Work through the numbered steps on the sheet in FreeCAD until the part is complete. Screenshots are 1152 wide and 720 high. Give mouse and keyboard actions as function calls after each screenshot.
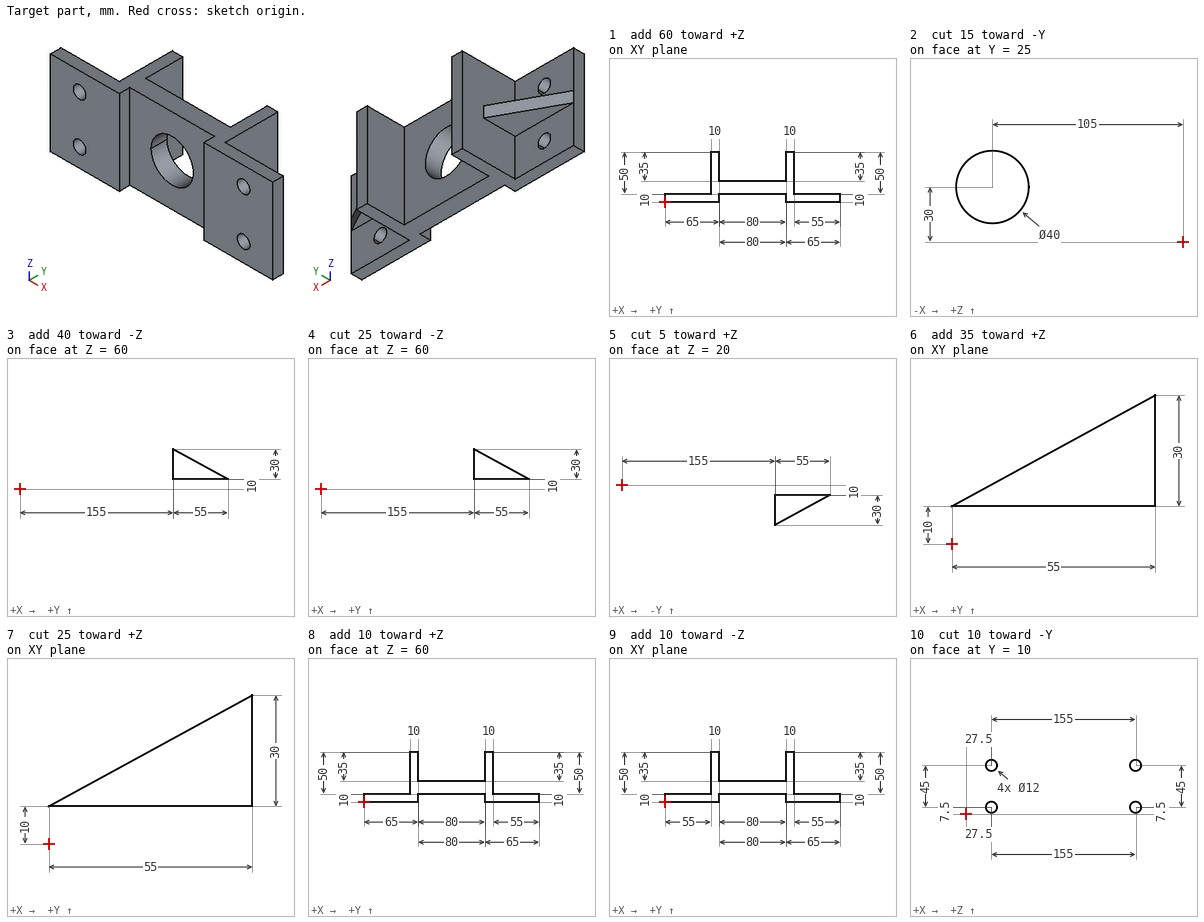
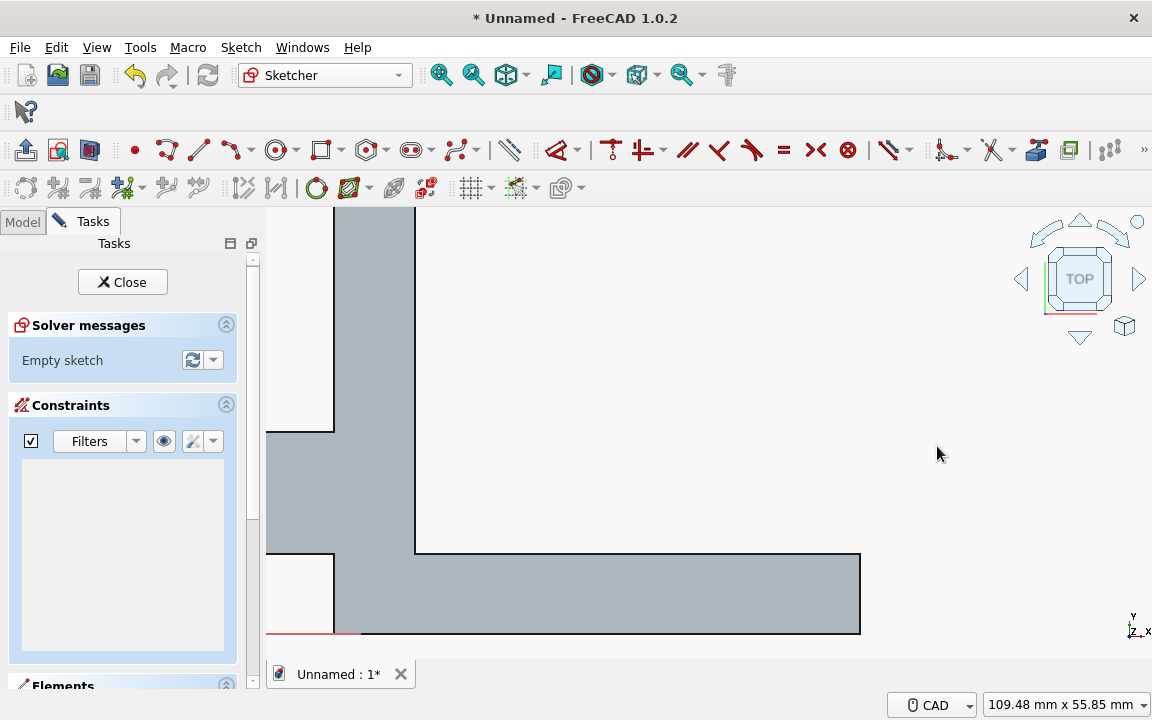
key(g)
key(m)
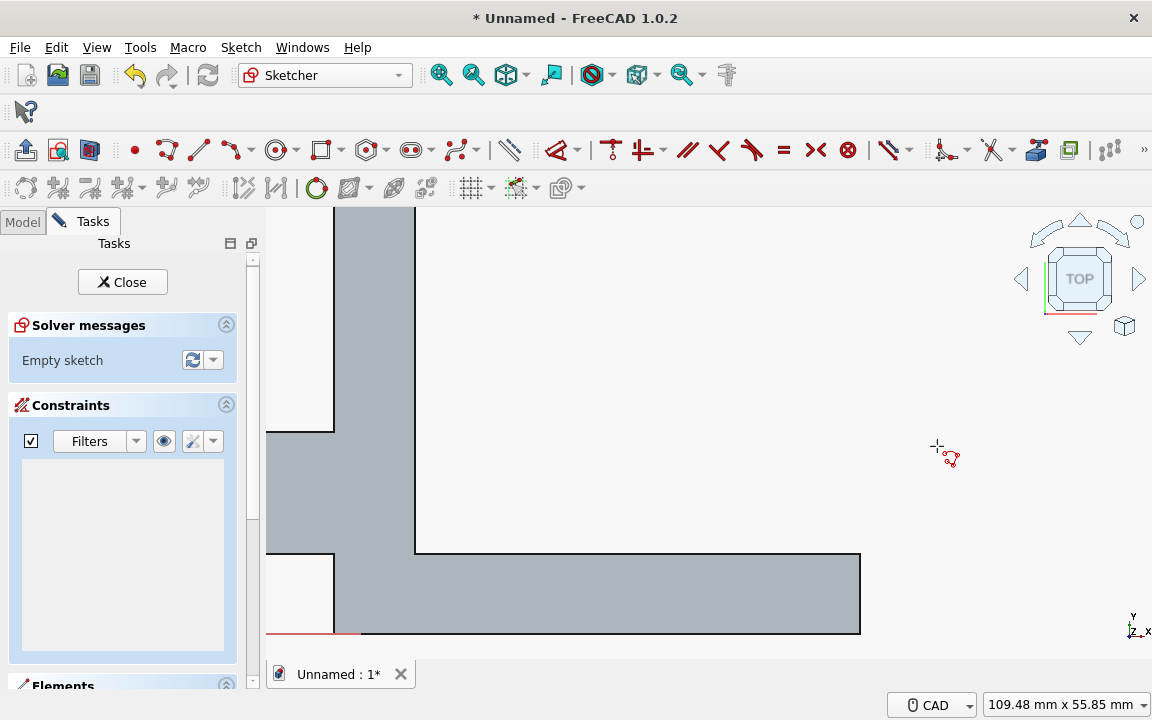
click(415, 554)
click(860, 554)
click(415, 311)
click(415, 555)
key(Escape)
key(Escape)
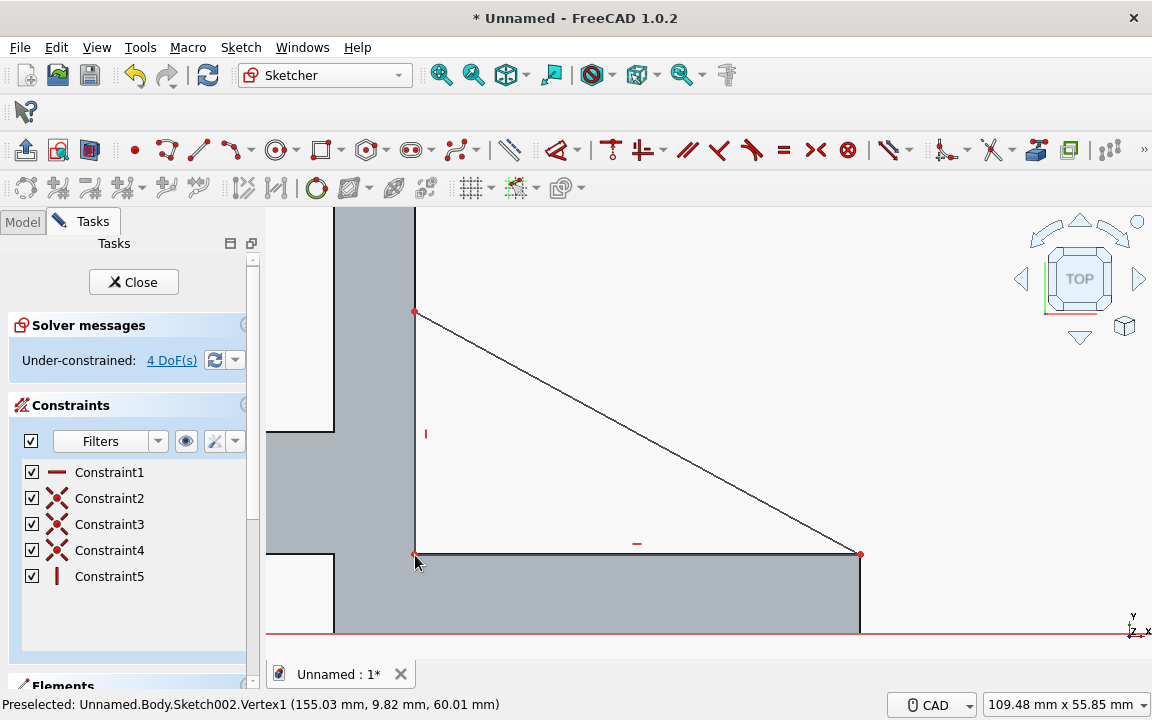
key(d)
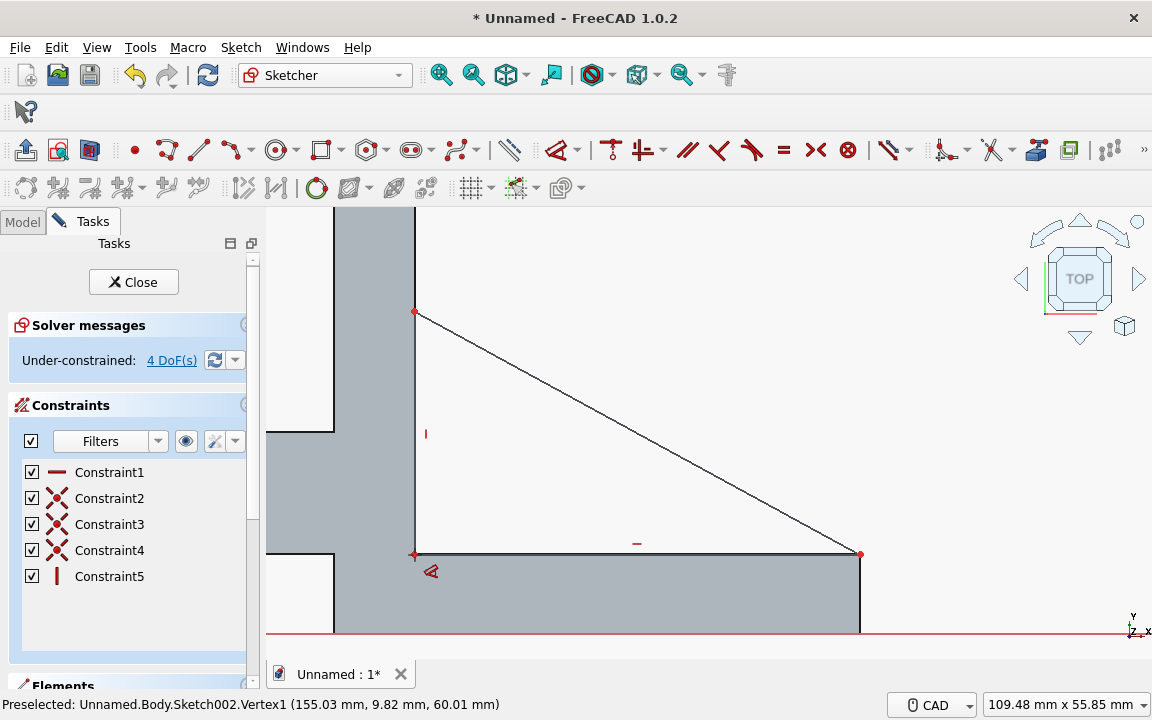
click(548, 555)
click(637, 589)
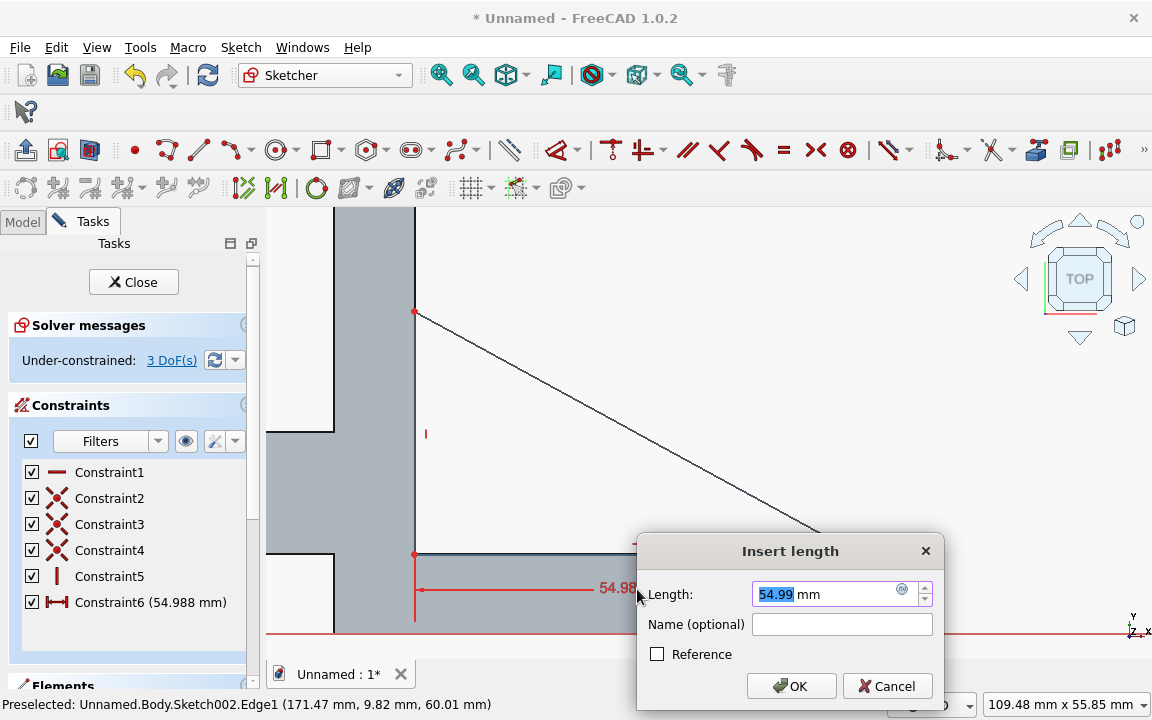
text(55)
key(Return)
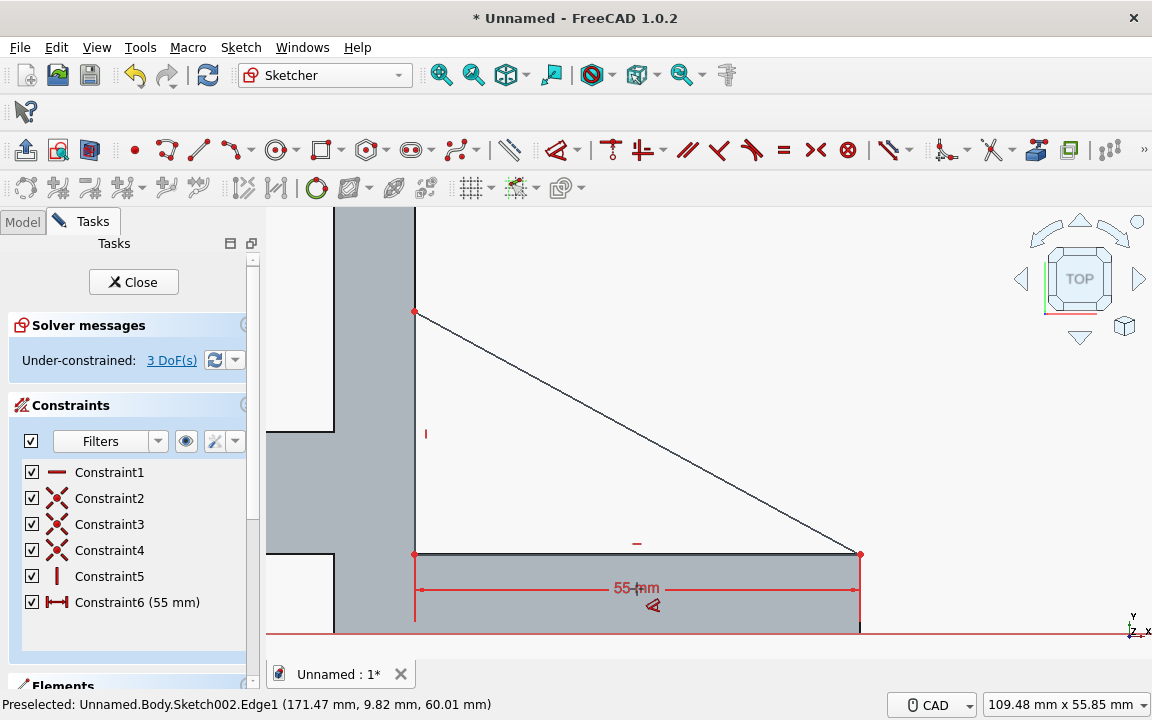
click(415, 385)
click(381, 433)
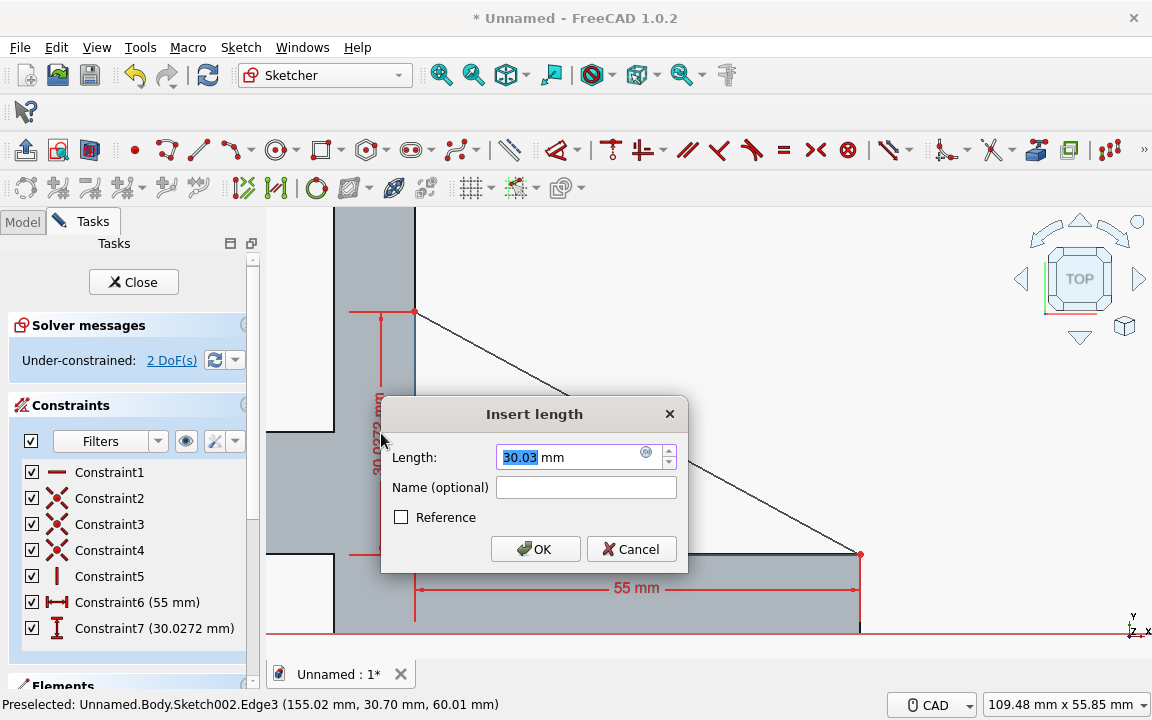
text(30)
key(Return)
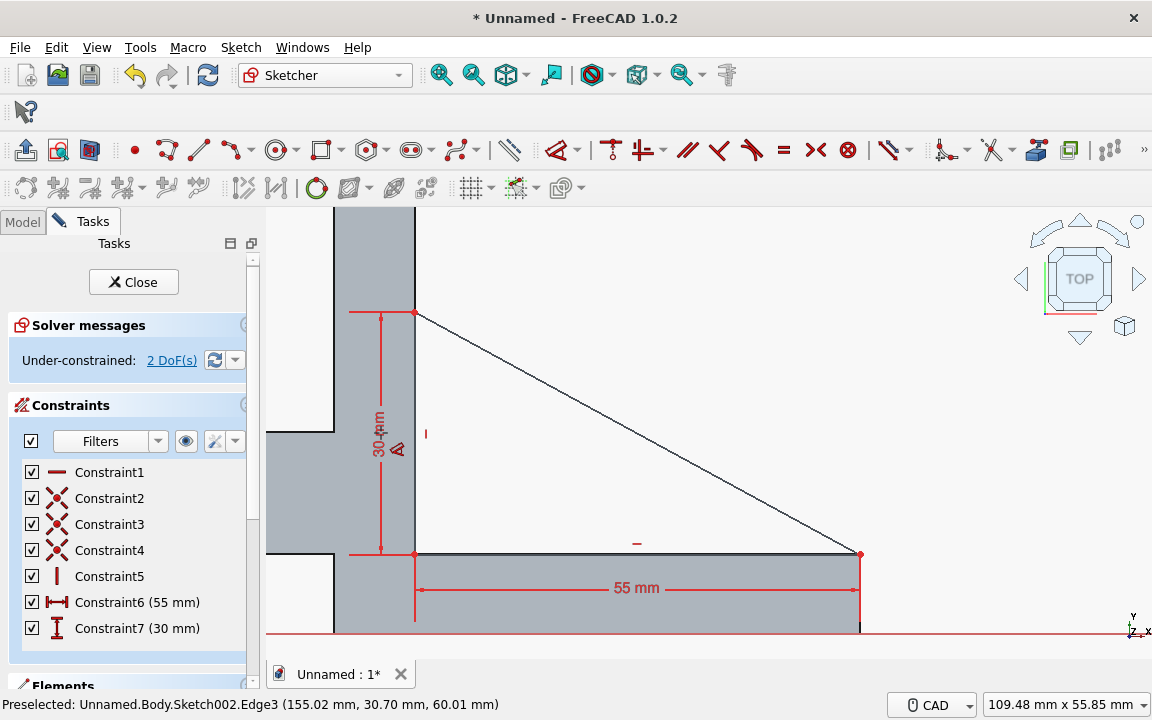
click(415, 555)
click(449, 593)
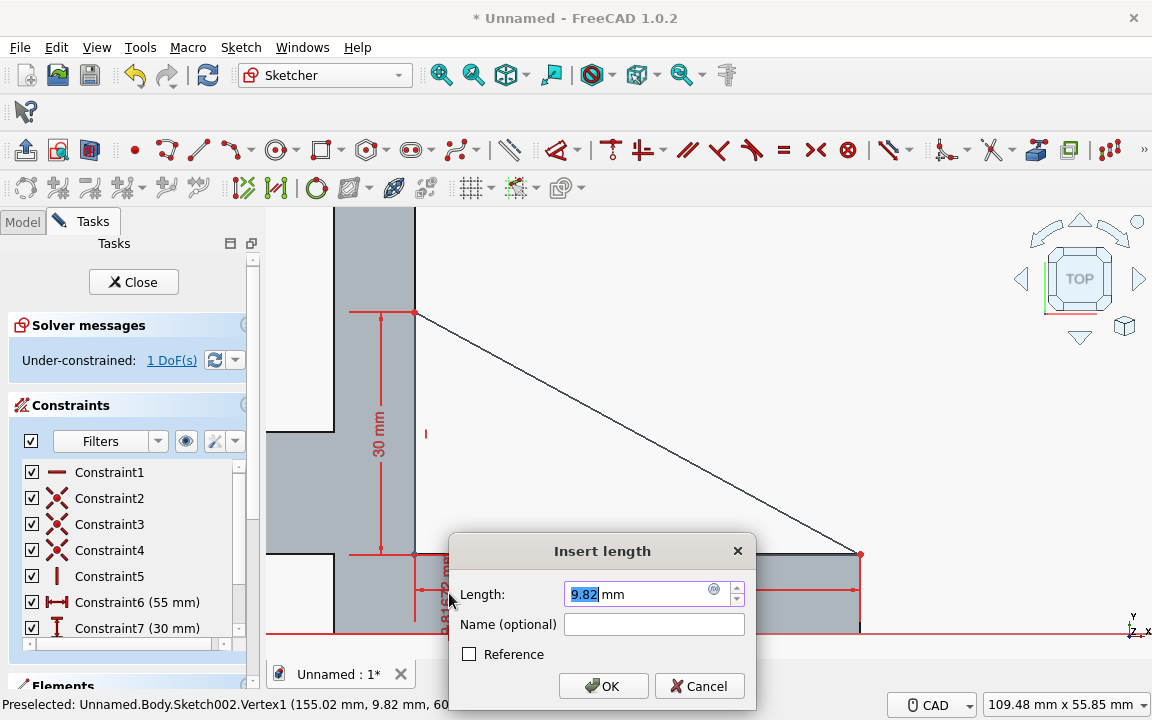
text(10)
key(Return)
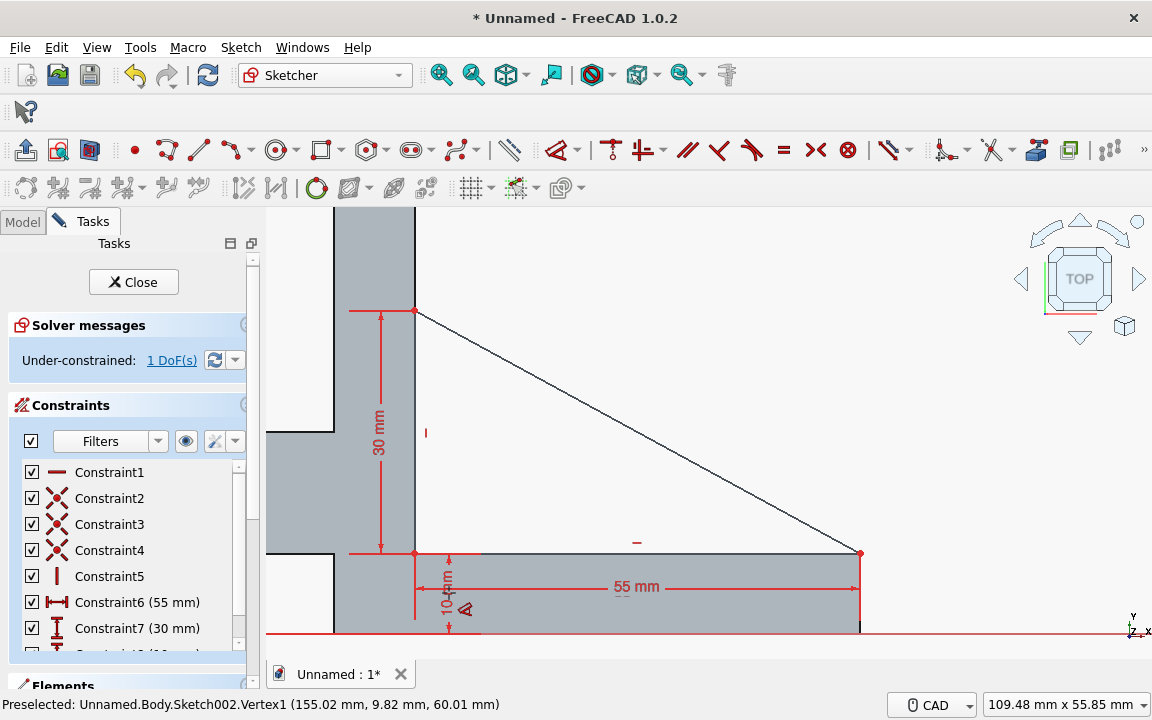
click(415, 554)
click(354, 520)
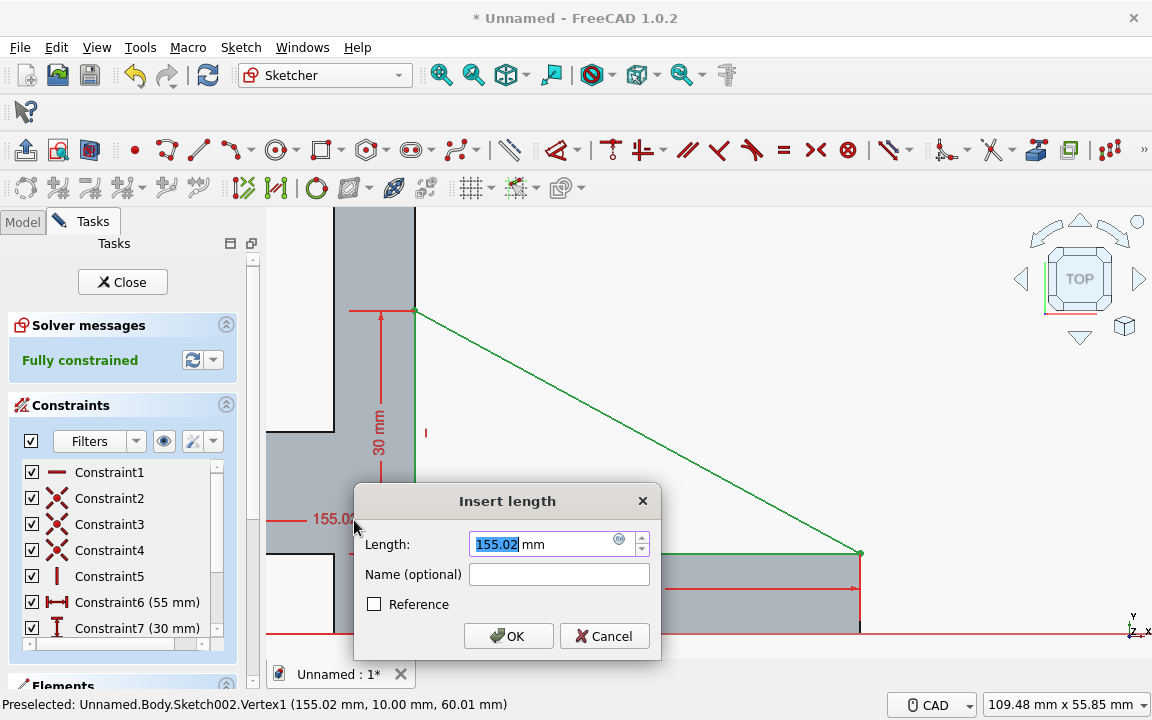
text(155)
key(Return)
key(Escape)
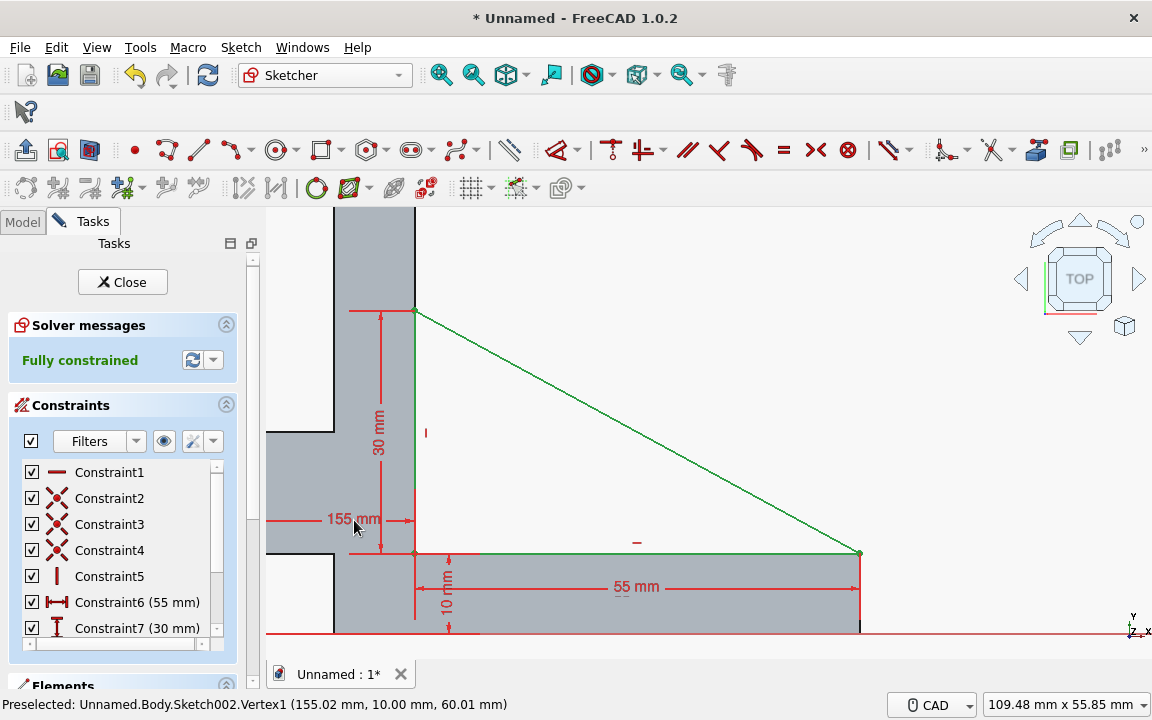
click(123, 282)